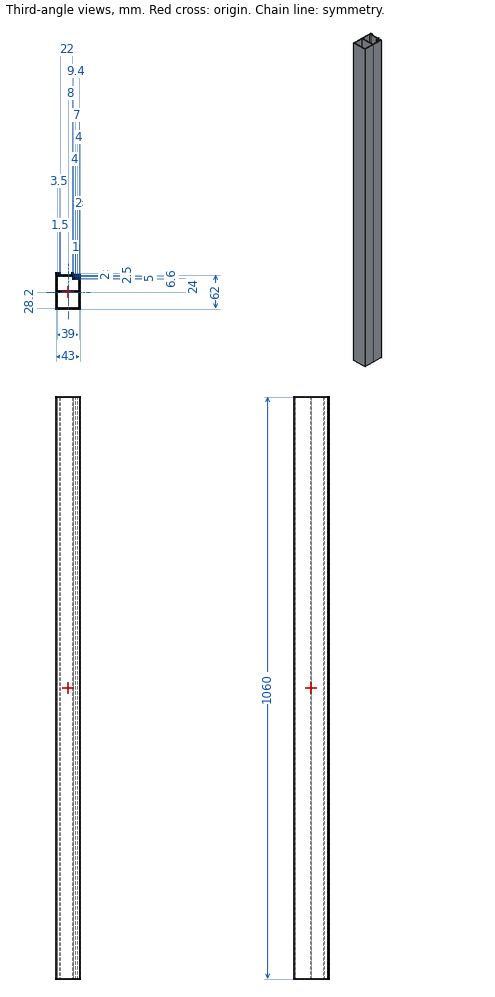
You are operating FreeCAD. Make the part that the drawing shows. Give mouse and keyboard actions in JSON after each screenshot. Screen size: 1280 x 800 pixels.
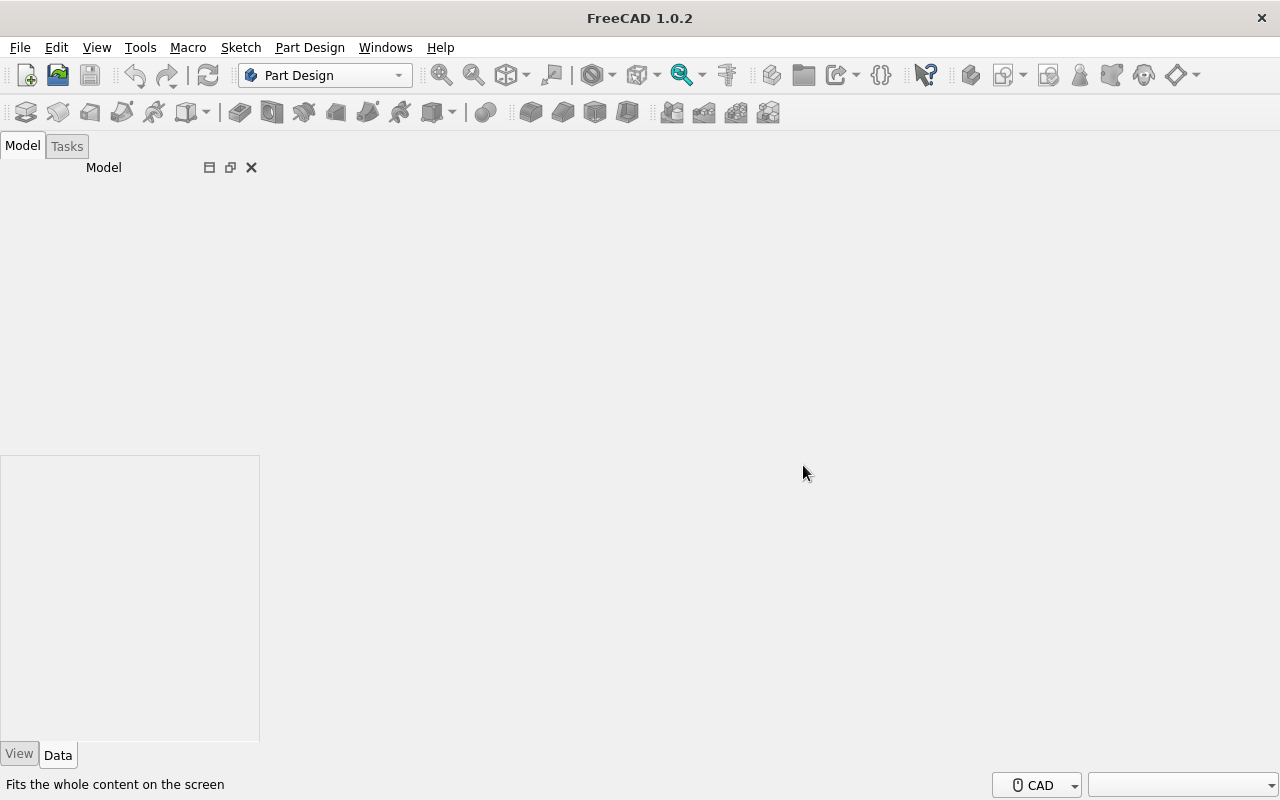
{"action": "left_click", "coordinate": [26, 76]}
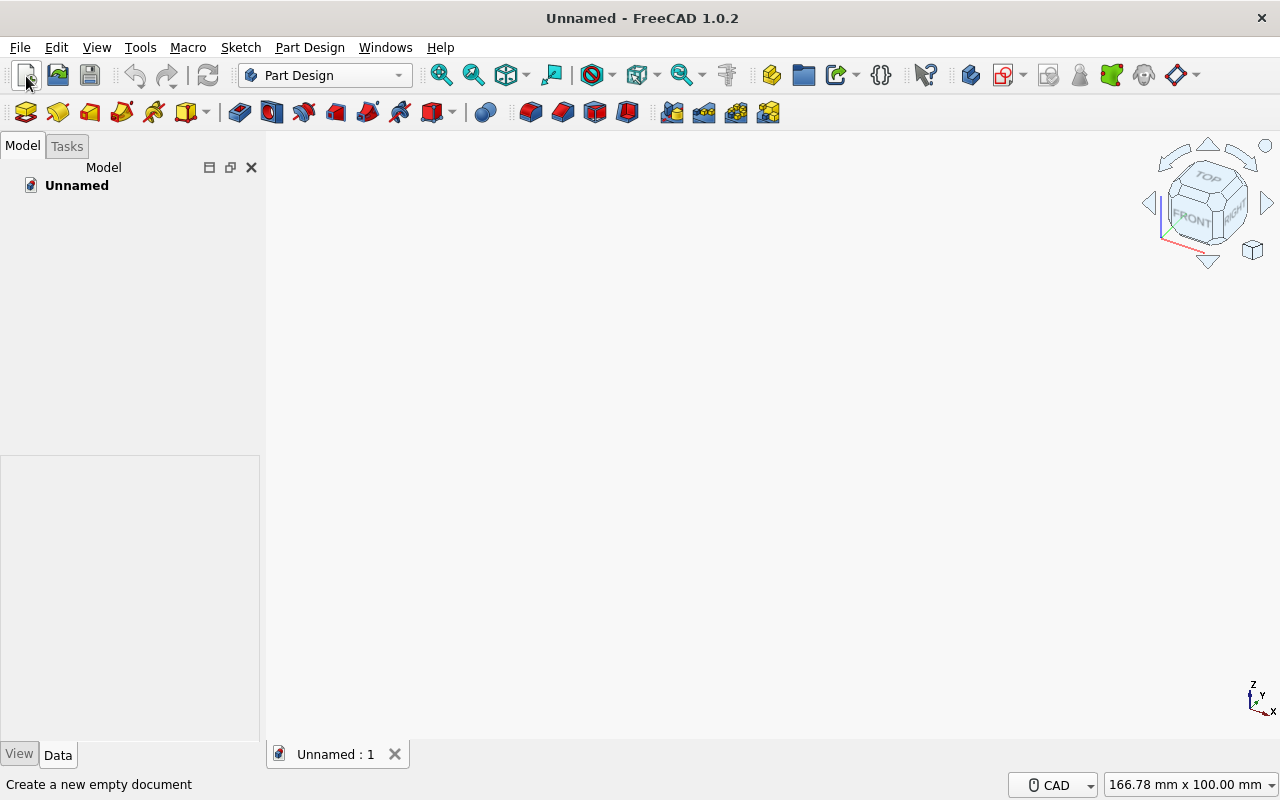
{"action": "left_click", "coordinate": [1004, 76]}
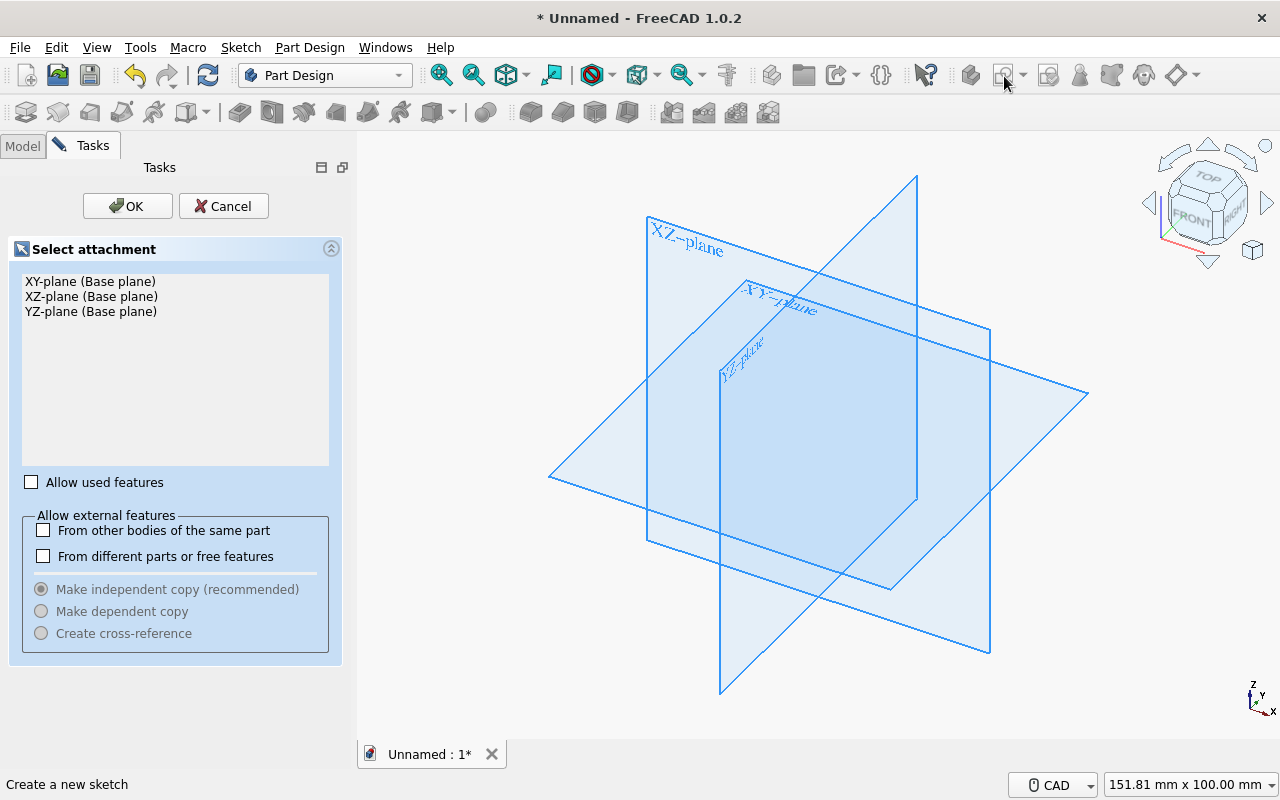
{"action": "left_click", "coordinate": [82, 282]}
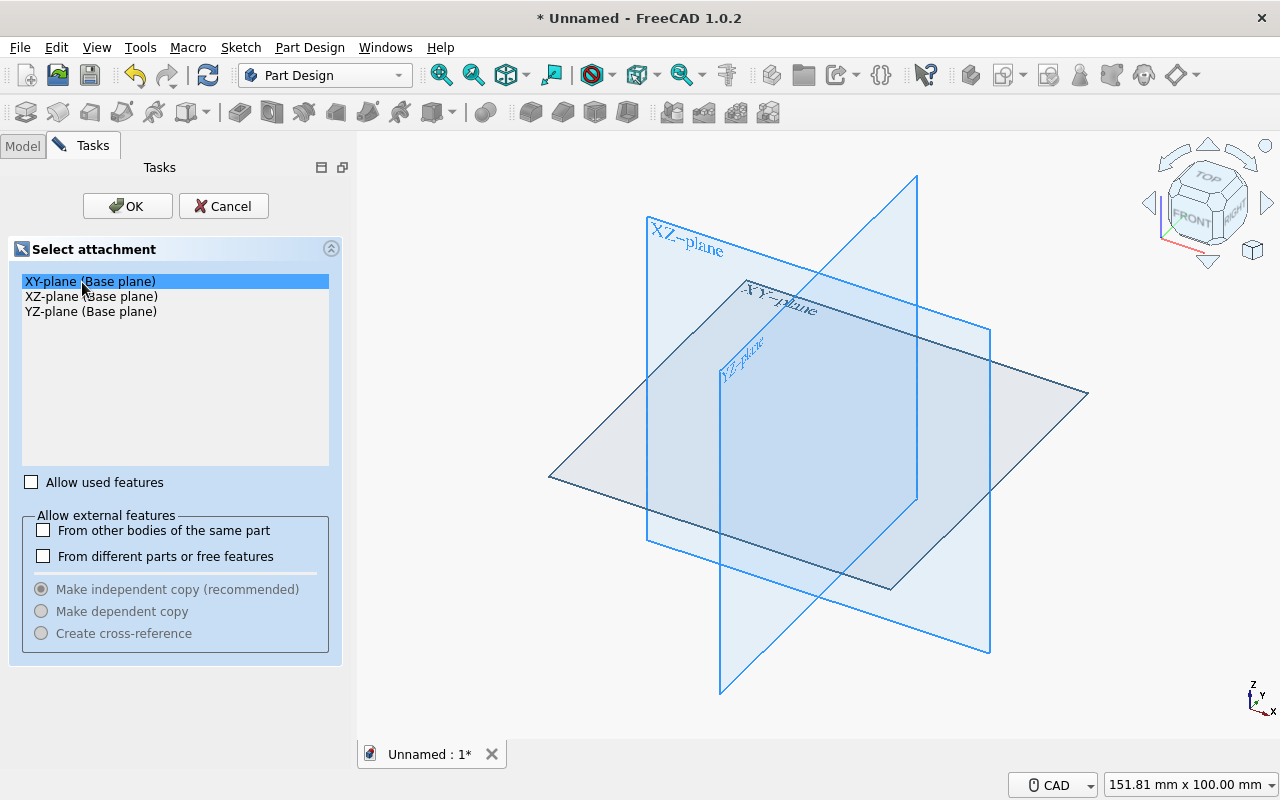
{"action": "left_click", "coordinate": [128, 206]}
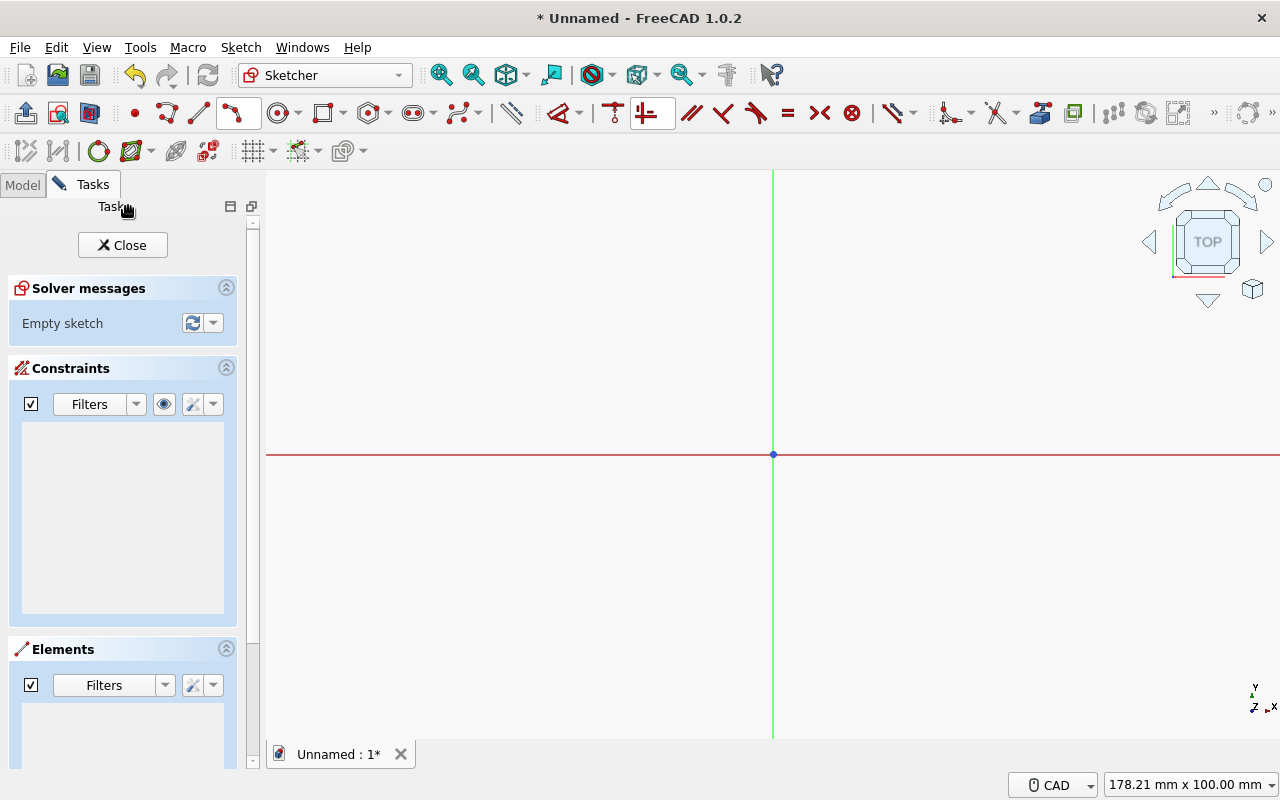
{"action": "left_click", "coordinate": [168, 114]}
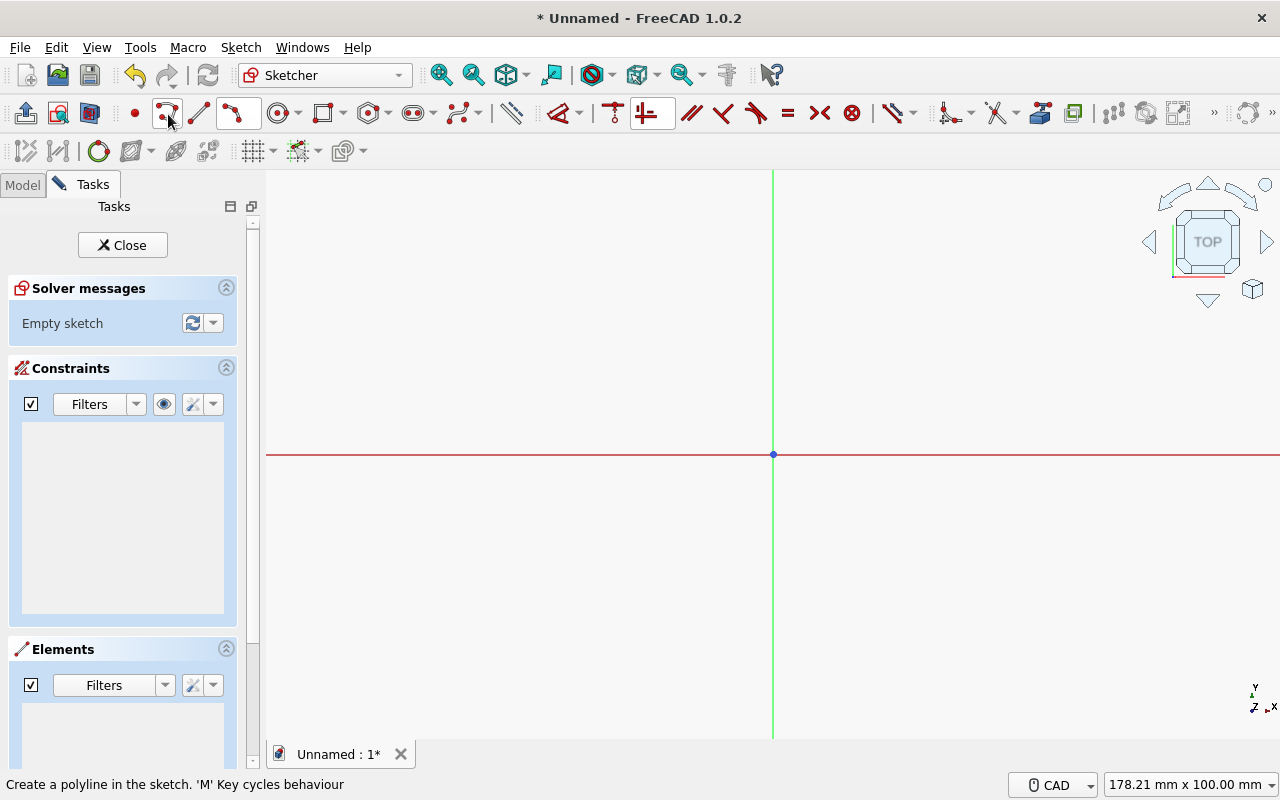
{"action": "left_click", "coordinate": [844, 318]}
{"action": "left_click", "coordinate": [844, 289]}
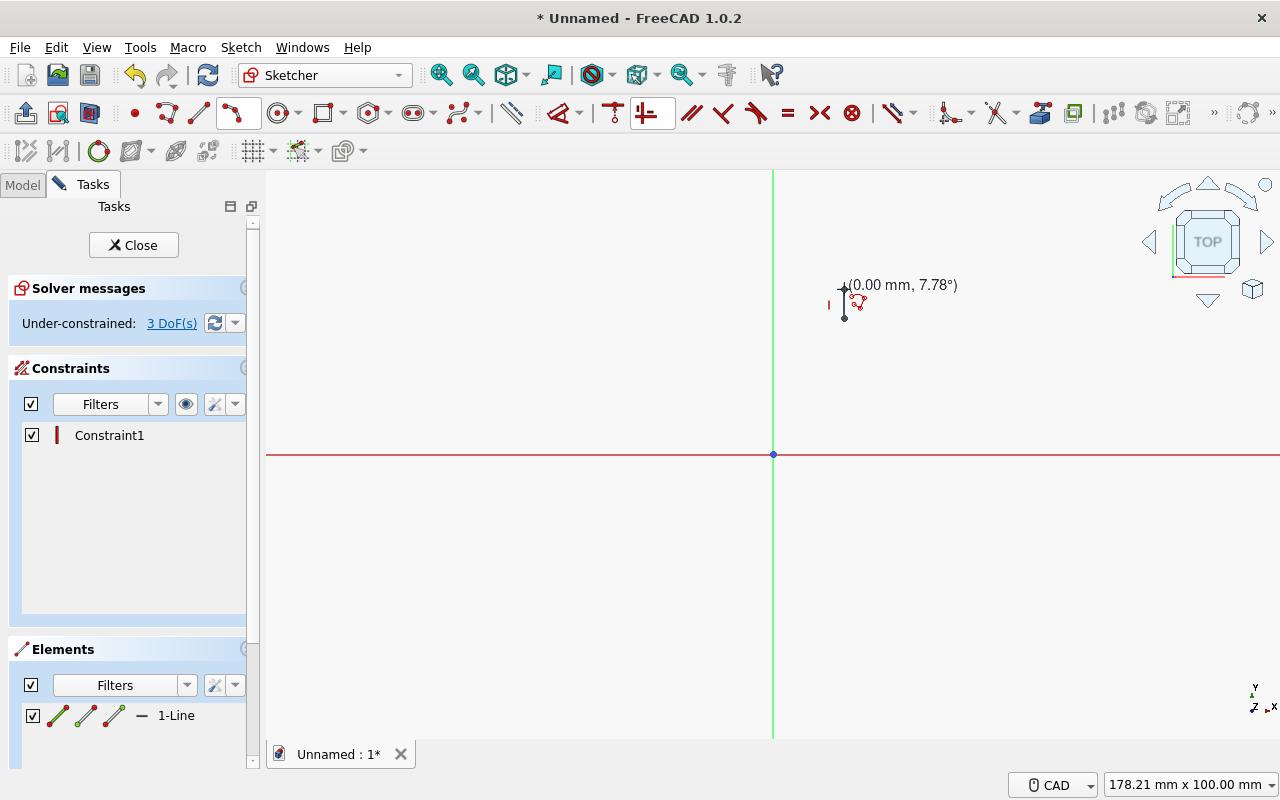
{"action": "scroll", "coordinate": [850, 289], "scroll_direction": "up", "scroll_amount": 6}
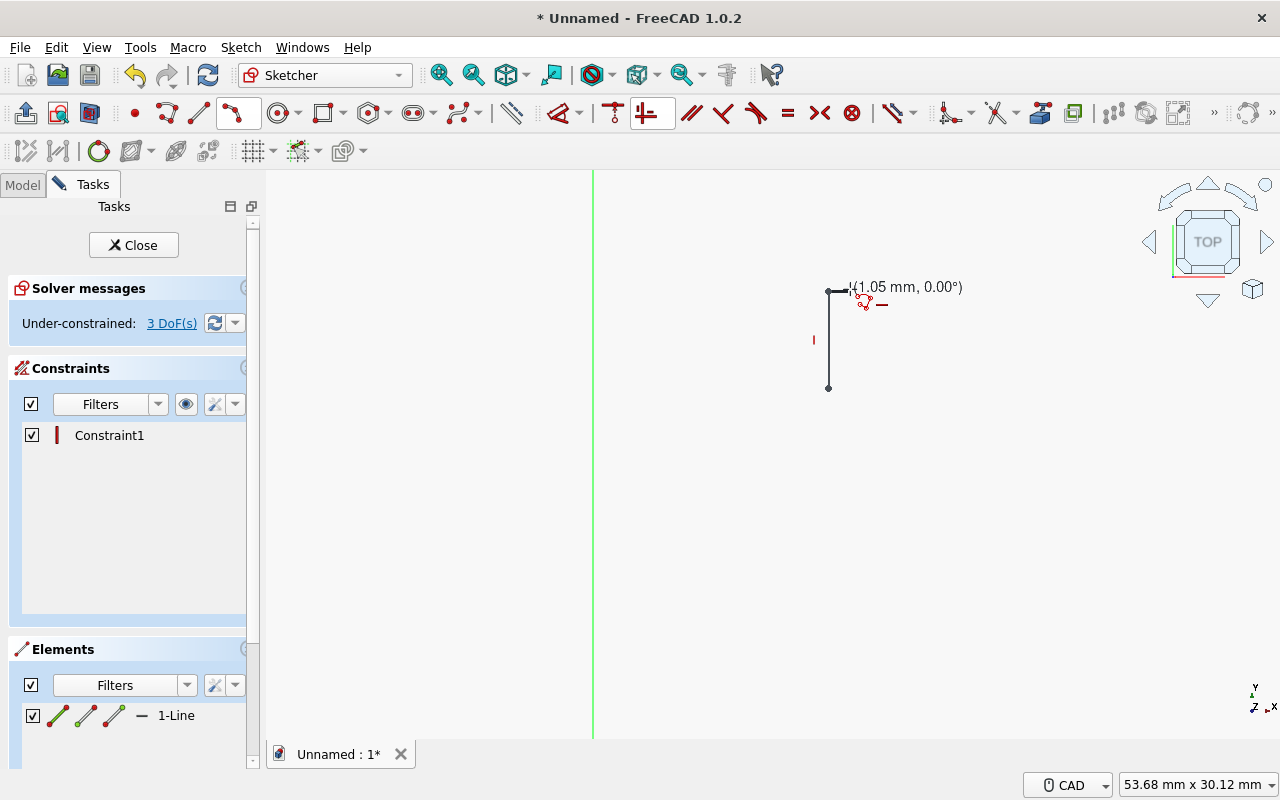
{"action": "left_click", "coordinate": [848, 289]}
{"action": "left_click", "coordinate": [848, 252]}
{"action": "left_click", "coordinate": [772, 252]}
{"action": "left_click", "coordinate": [772, 205]}
{"action": "left_click", "coordinate": [744, 205]}
{"action": "left_click", "coordinate": [744, 252]}
{"action": "left_click", "coordinate": [329, 252]}
{"action": "left_click", "coordinate": [329, 205]}
{"action": "left_click", "coordinate": [300, 205]}
{"action": "left_click", "coordinate": [300, 252]}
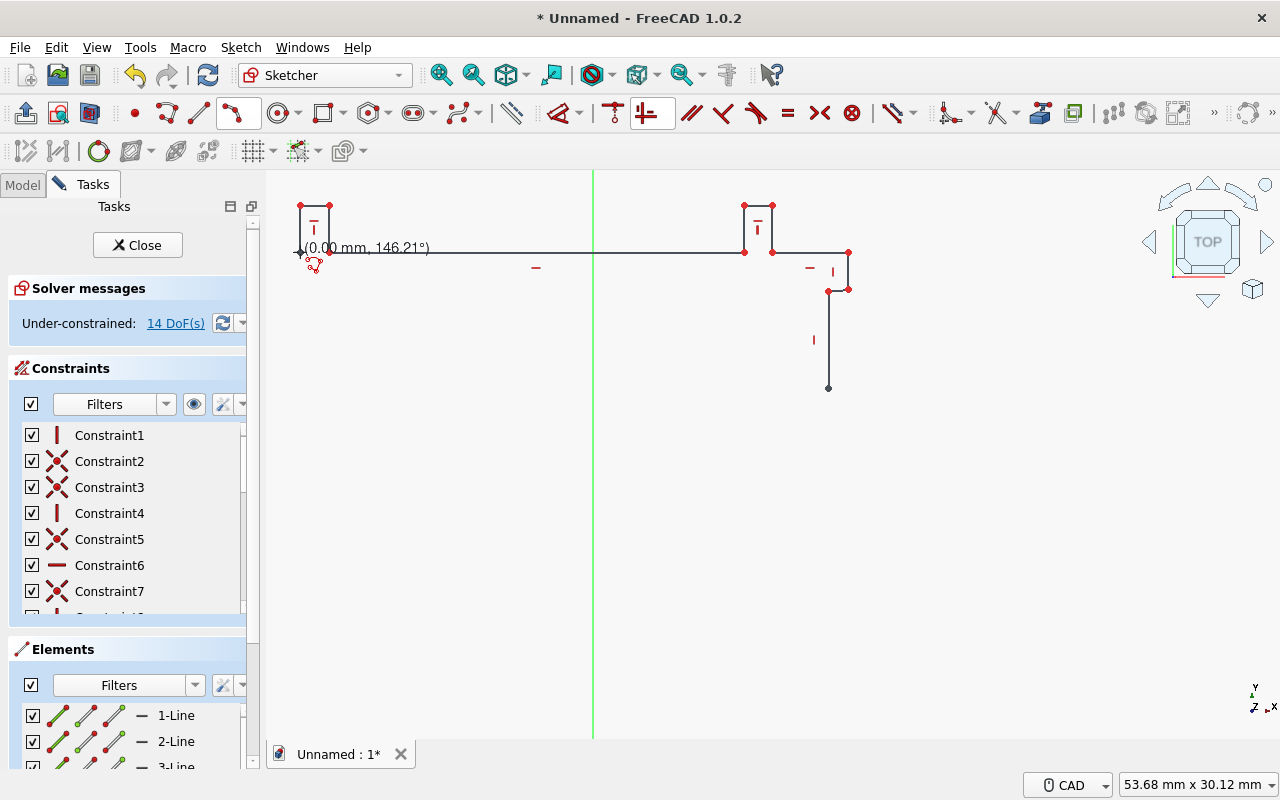
{"action": "scroll", "coordinate": [753, 299], "scroll_direction": "down", "scroll_amount": 6}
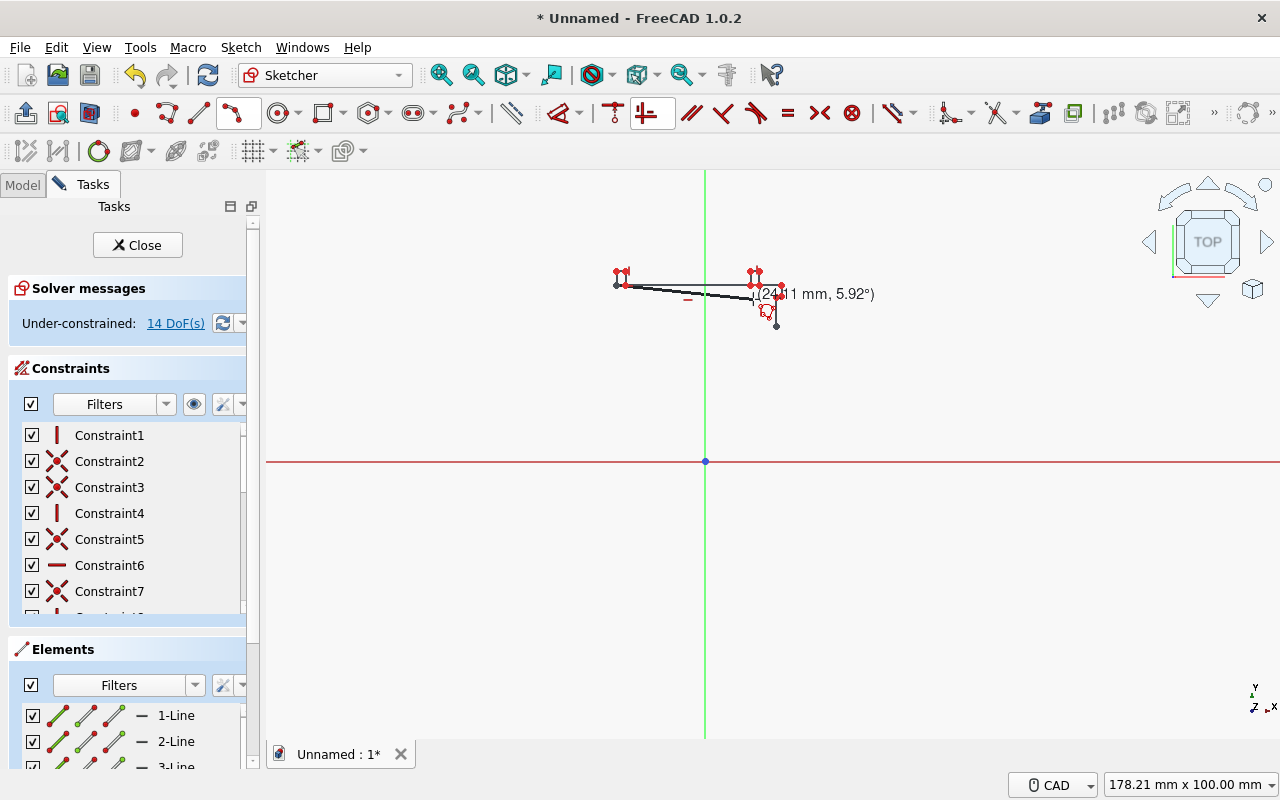
{"action": "left_click", "coordinate": [597, 285]}
{"action": "left_click", "coordinate": [597, 271]}
{"action": "left_click", "coordinate": [583, 271]}
{"action": "left_click", "coordinate": [583, 638]}
{"action": "left_click", "coordinate": [827, 638]}
{"action": "left_click", "coordinate": [827, 285]}
{"action": "left_click", "coordinate": [805, 285]}